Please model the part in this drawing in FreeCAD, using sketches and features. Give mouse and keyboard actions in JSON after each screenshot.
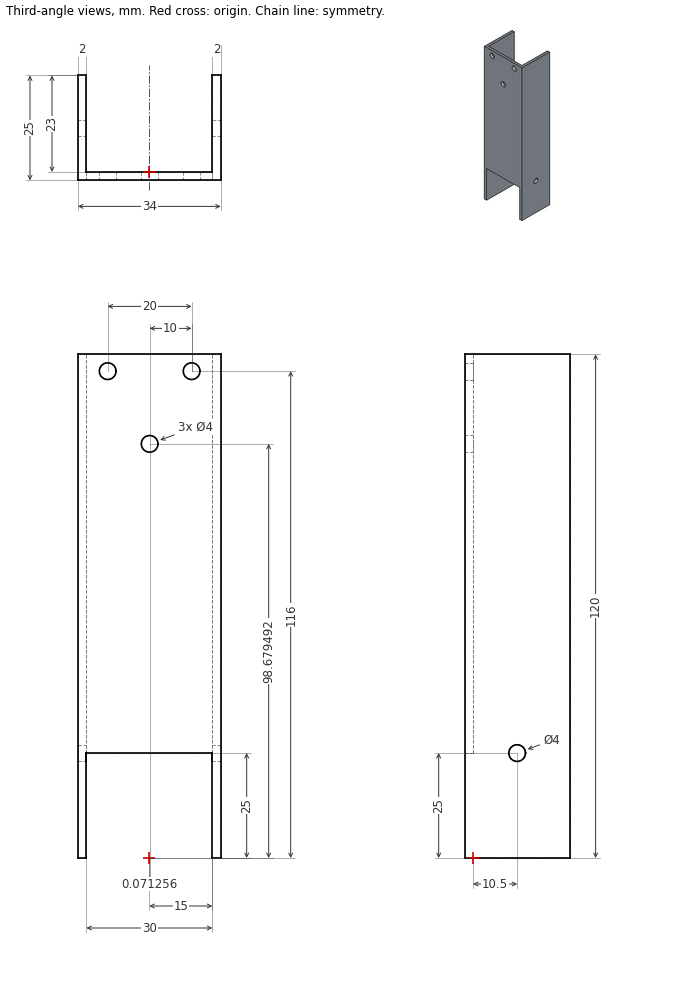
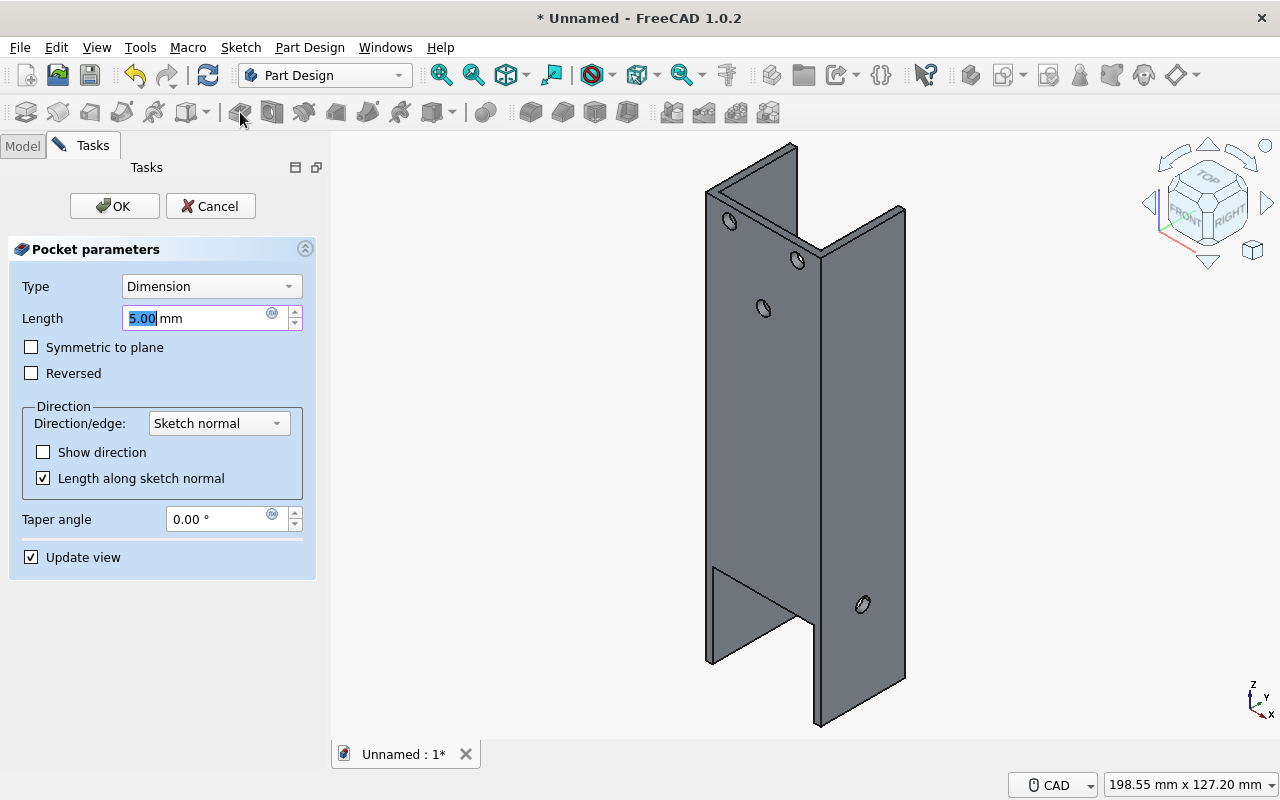
{"action": "left_click", "coordinate": [212, 286]}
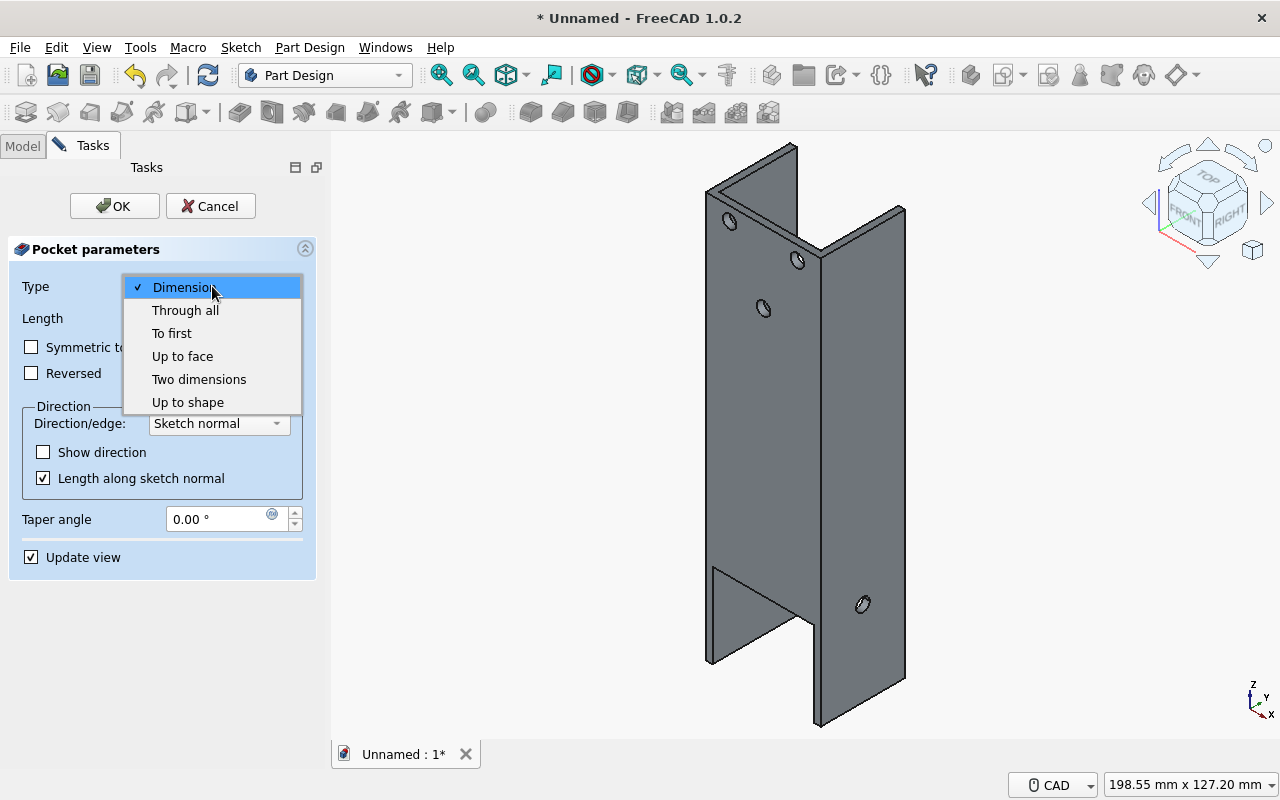
{"action": "left_click", "coordinate": [212, 310]}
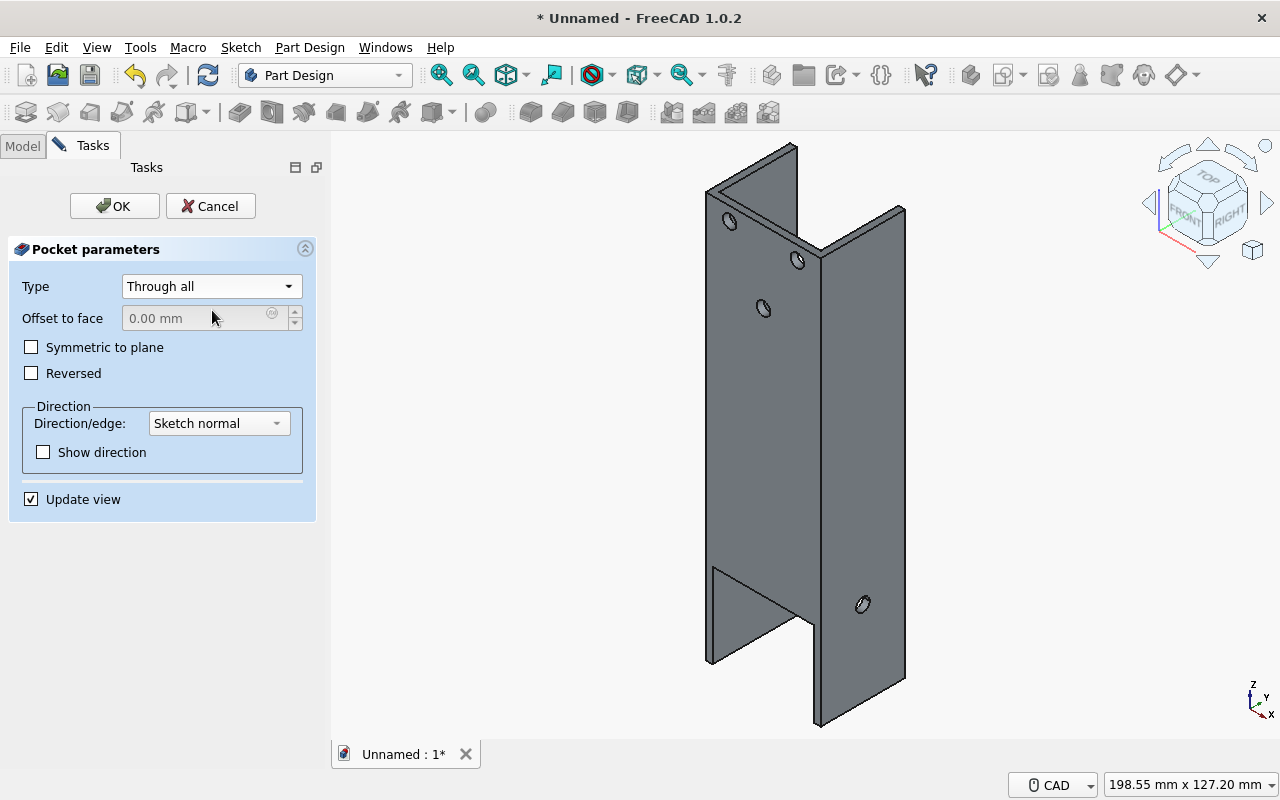
{"action": "left_click", "coordinate": [115, 206]}